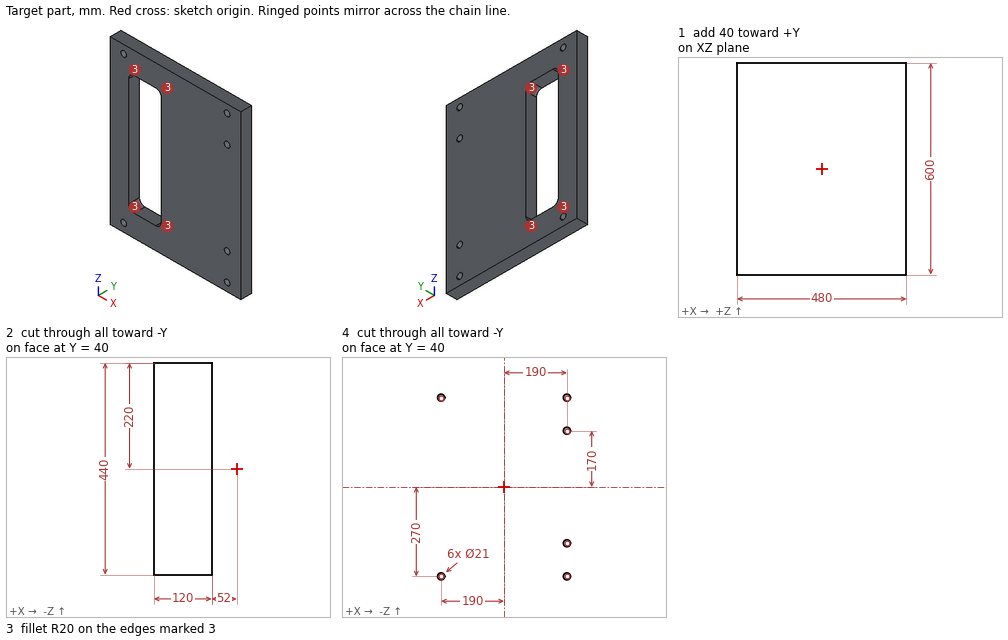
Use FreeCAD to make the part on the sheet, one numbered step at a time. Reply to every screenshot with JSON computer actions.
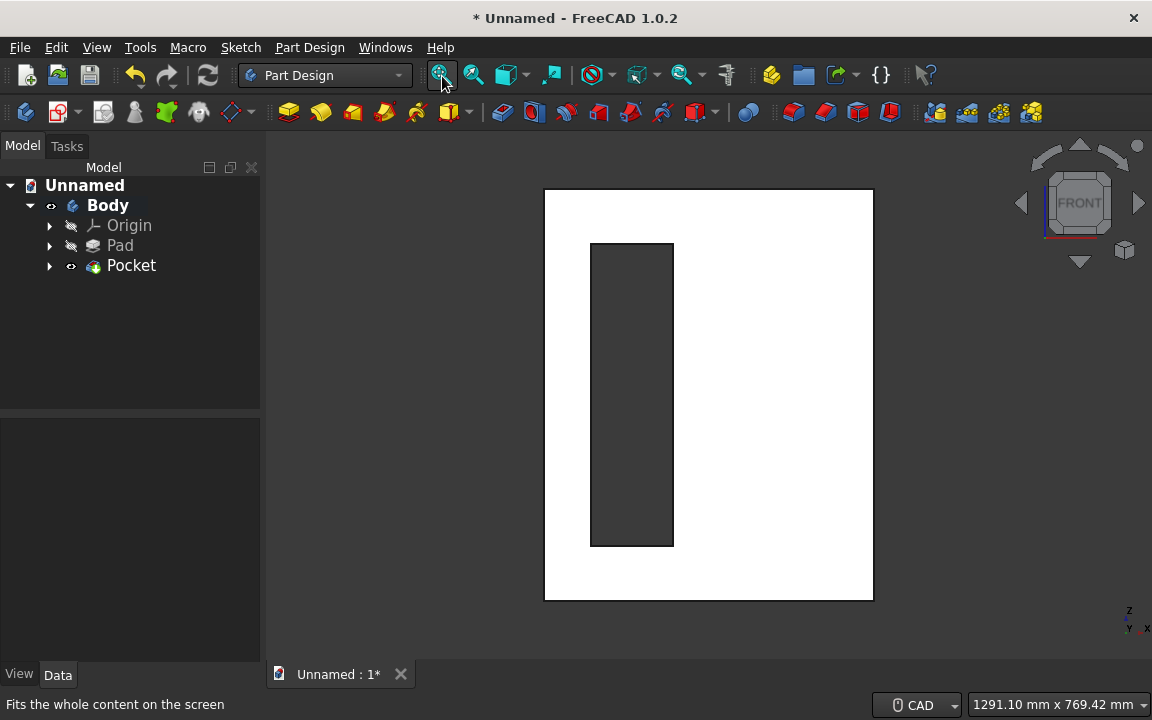
{"action": "key", "text": "3"}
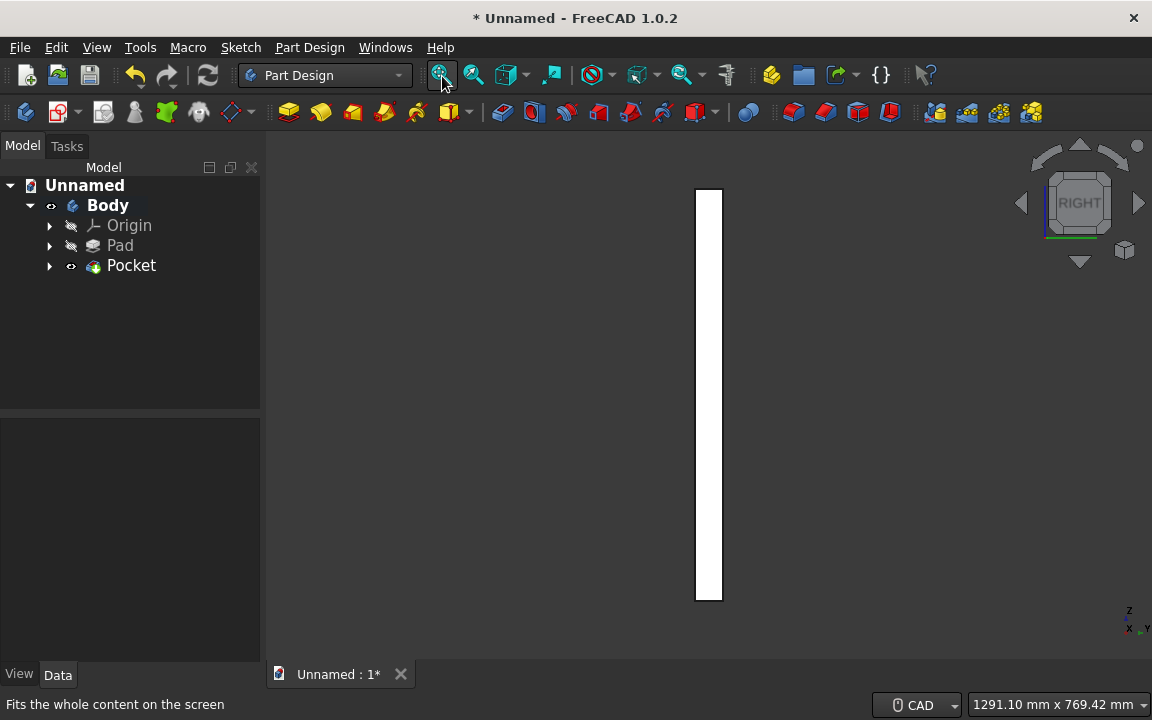
{"action": "key", "text": "5"}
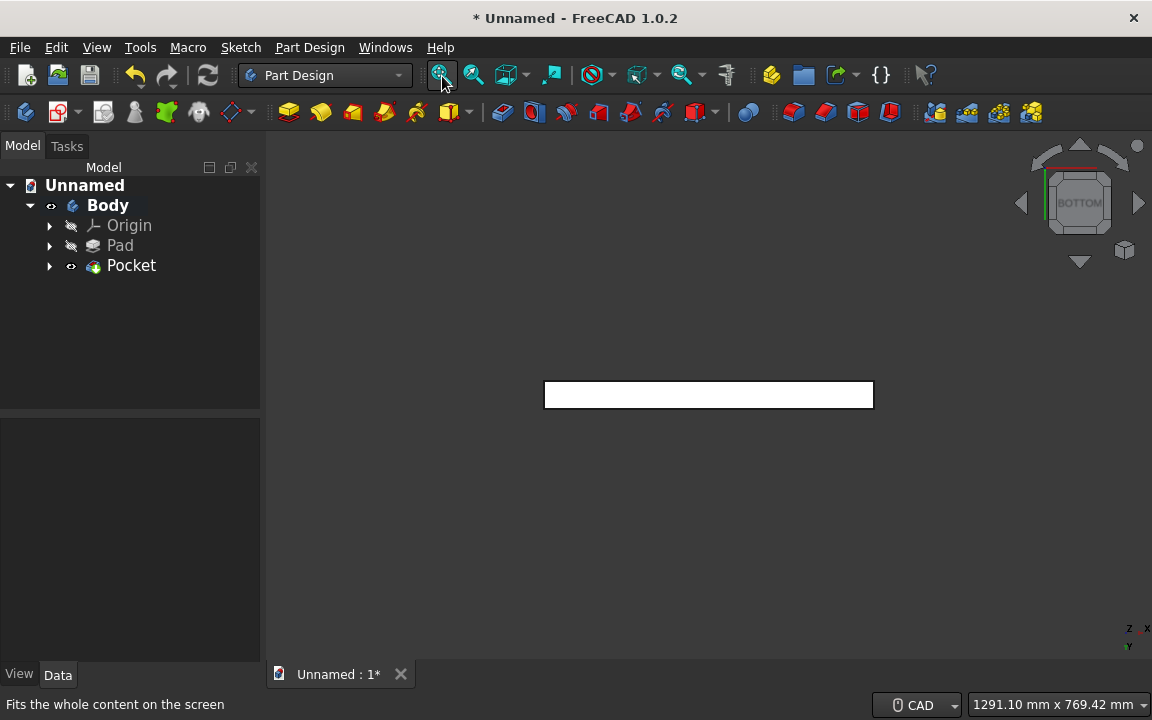
{"action": "left_click", "coordinate": [442, 76]}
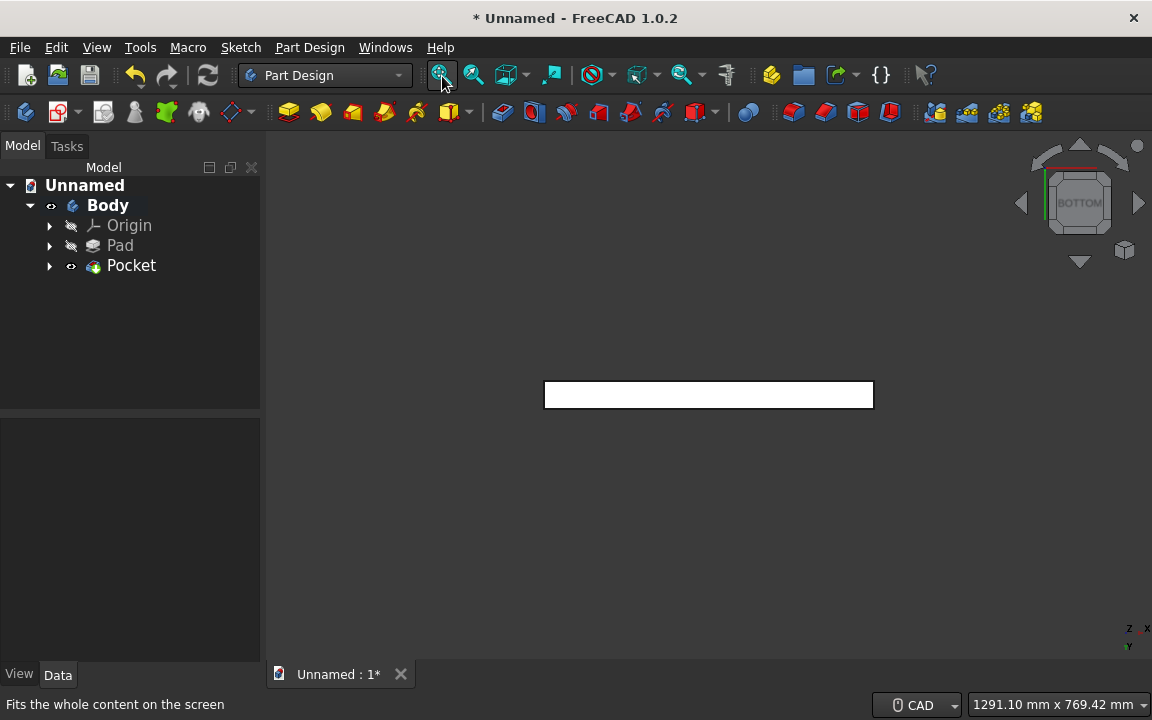
{"action": "key", "text": "4"}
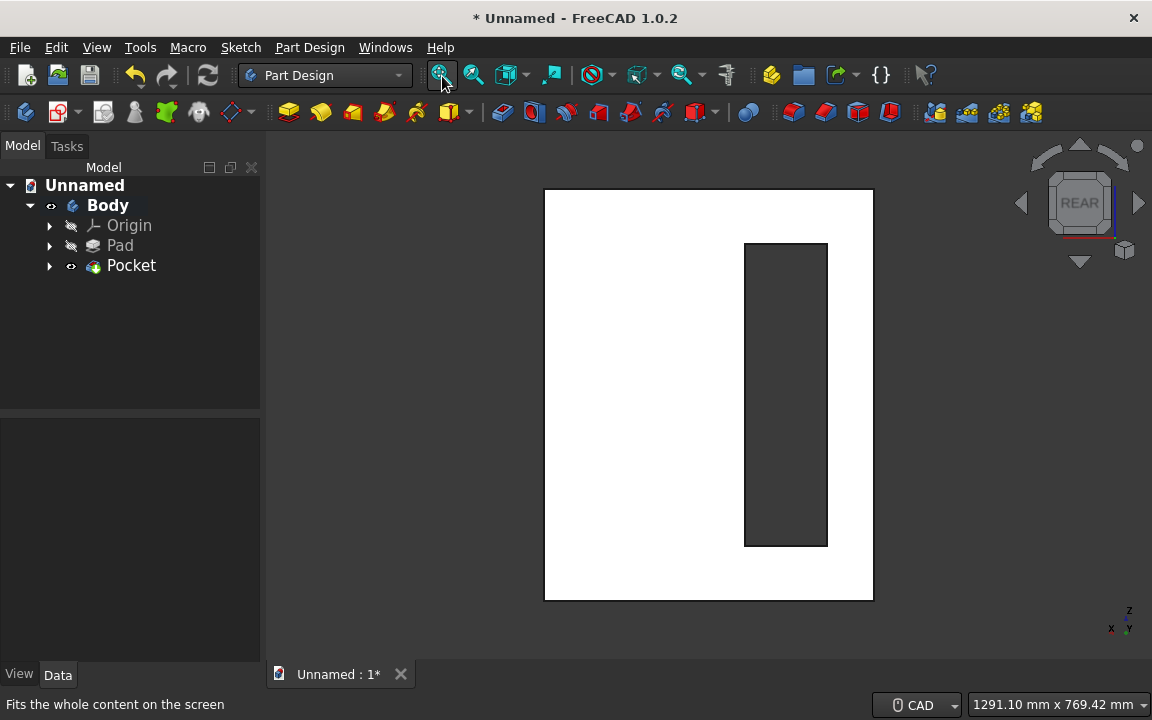
{"action": "key", "text": "6"}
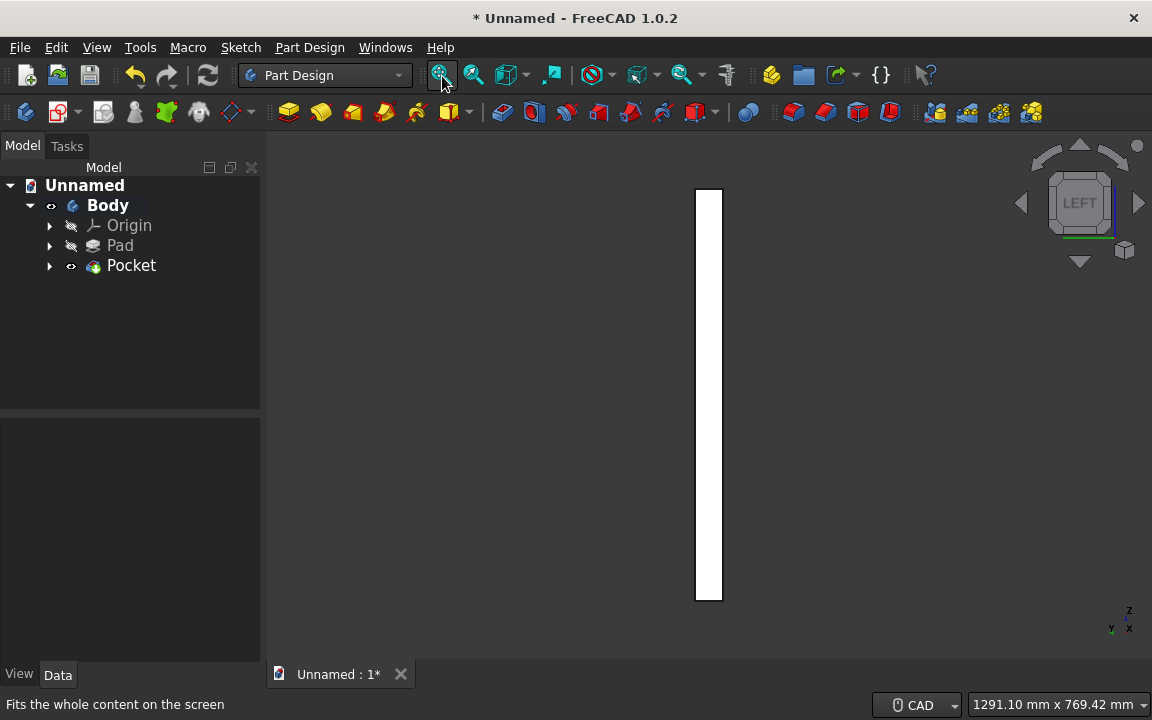
{"action": "key", "text": "v 3"}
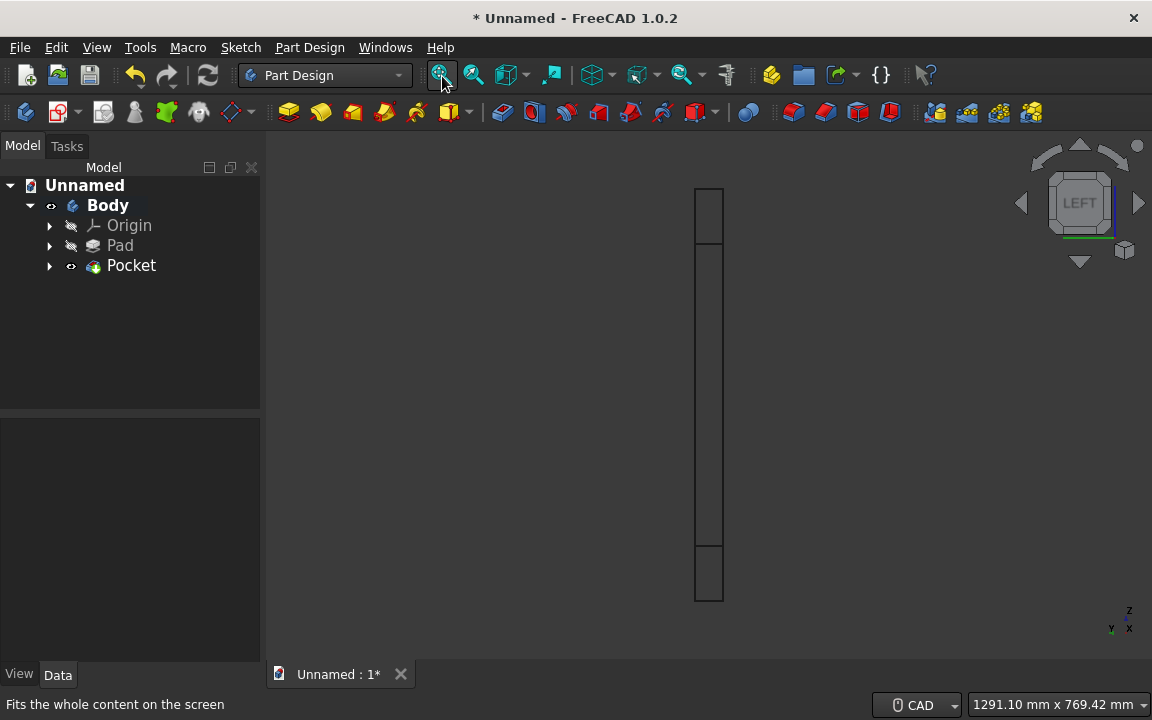
{"action": "key", "text": "0"}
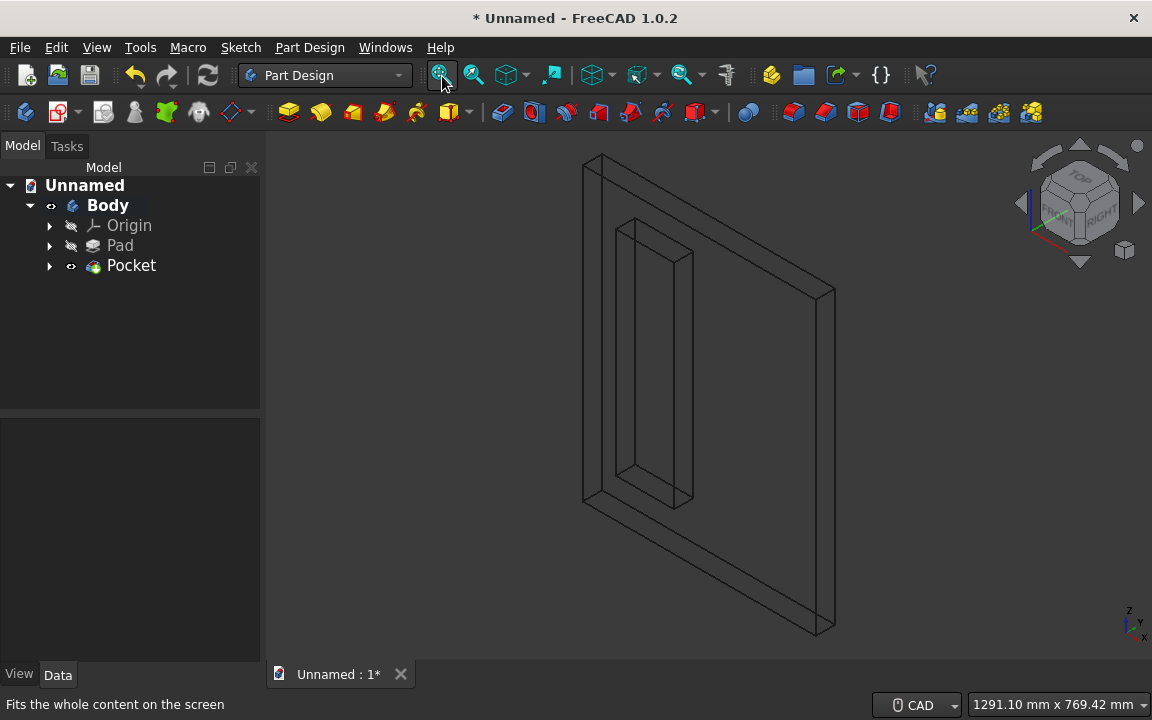
{"action": "left_click", "coordinate": [684, 503]}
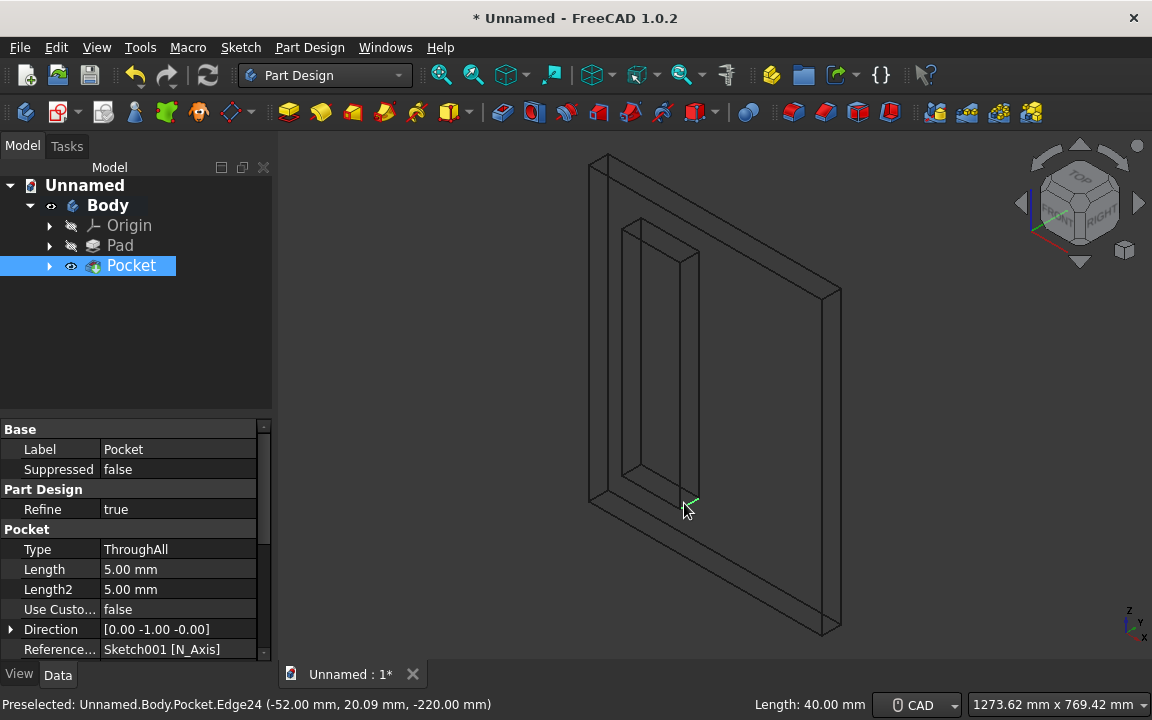
{"action": "left_click", "coordinate": [690, 256], "text": "ctrl"}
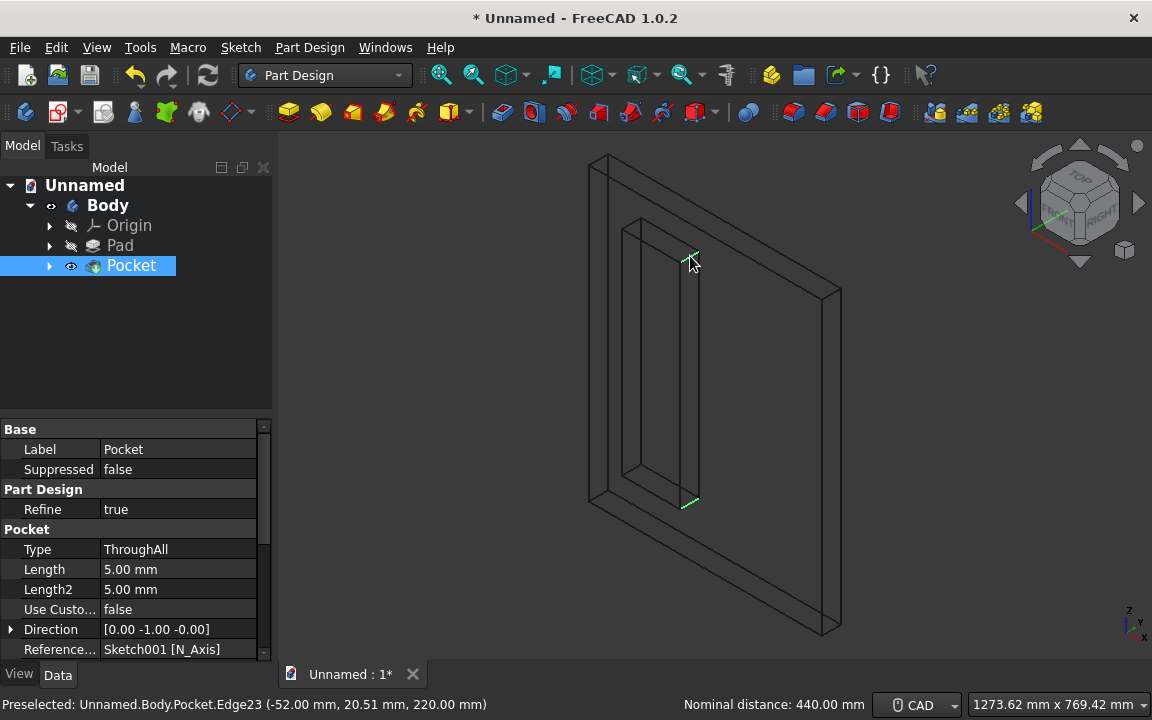
{"action": "left_click", "coordinate": [632, 223], "text": "ctrl"}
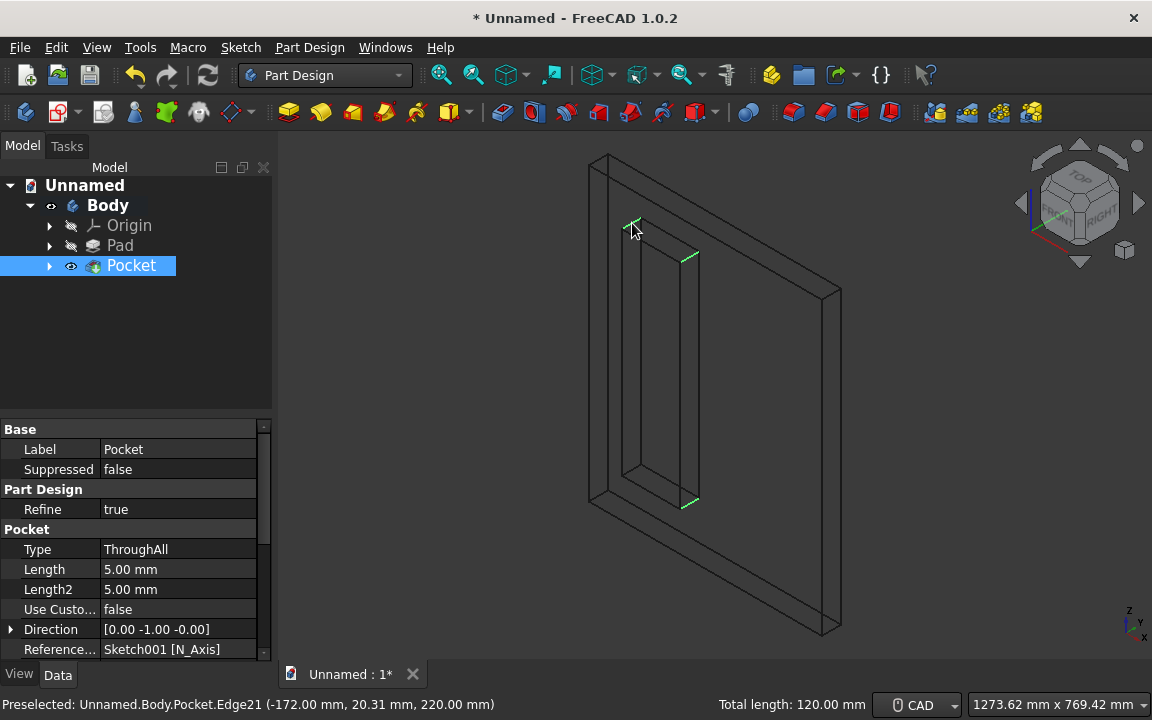
{"action": "left_click", "coordinate": [632, 469], "text": "ctrl"}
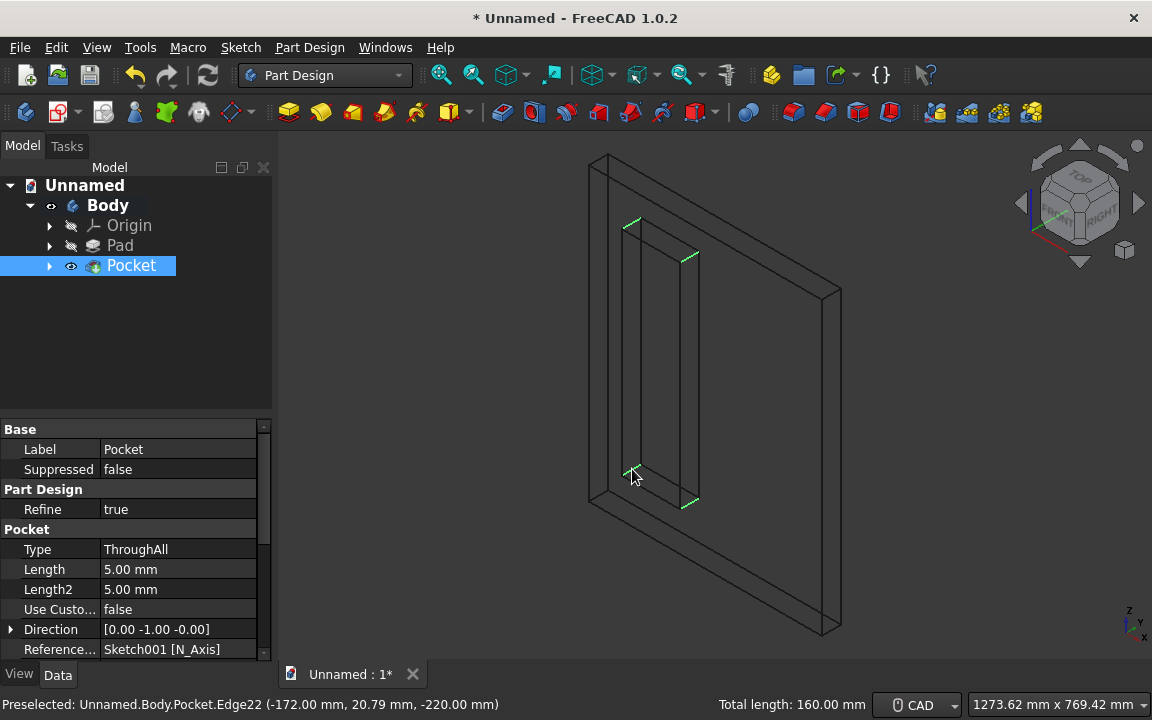
{"action": "key", "text": "v 1"}